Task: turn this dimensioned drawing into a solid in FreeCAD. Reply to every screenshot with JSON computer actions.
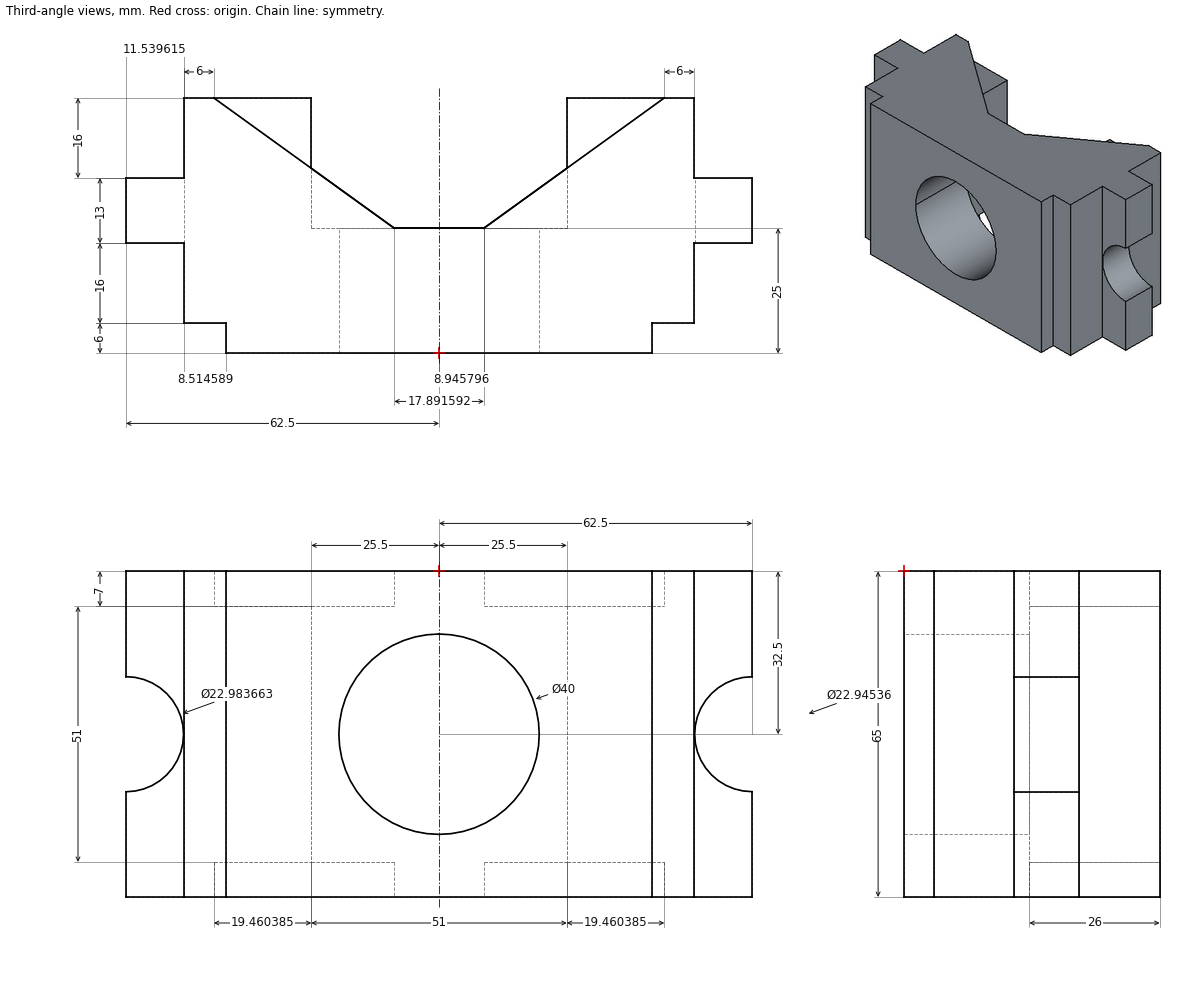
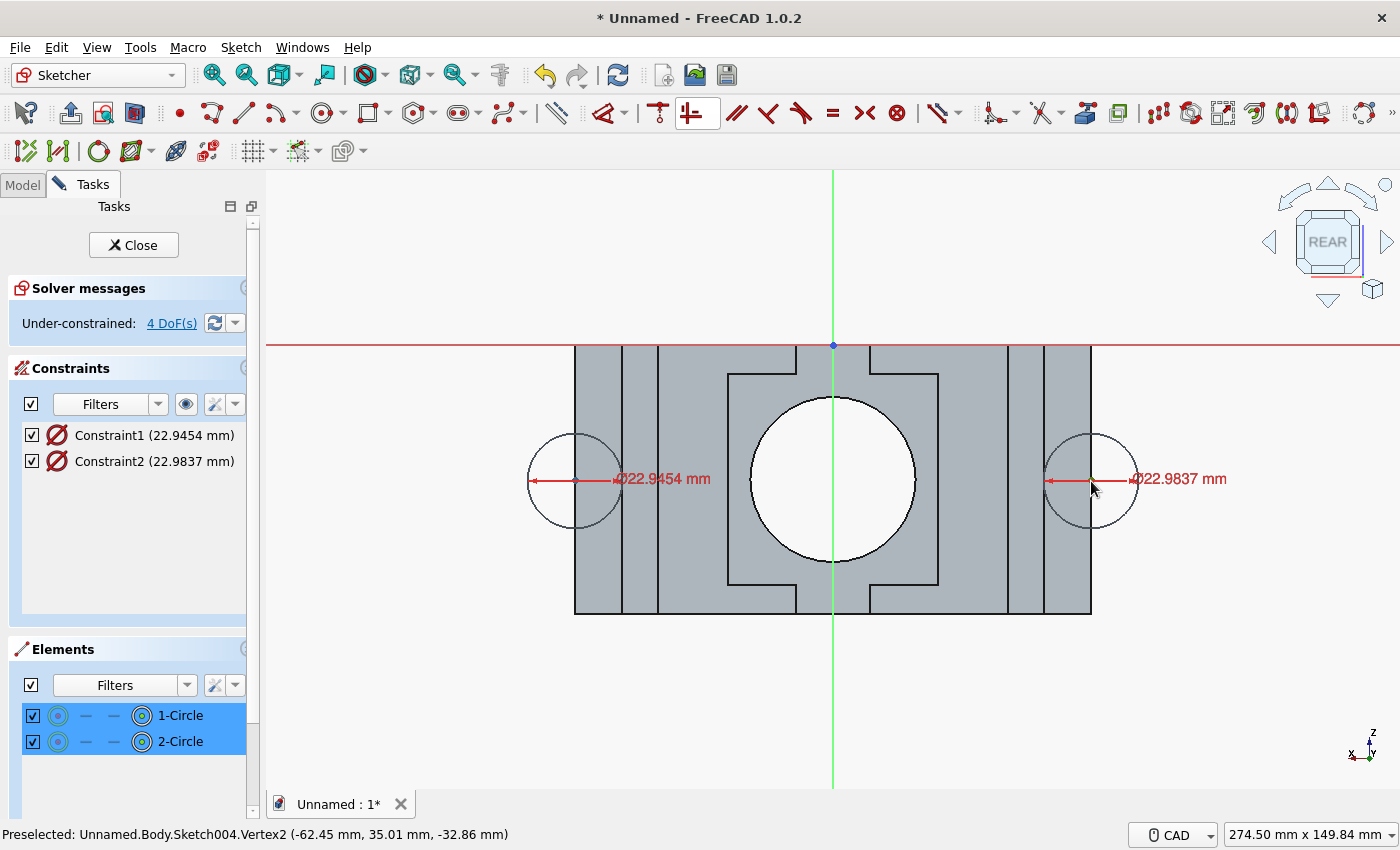
{"action": "left_click", "coordinate": [833, 721]}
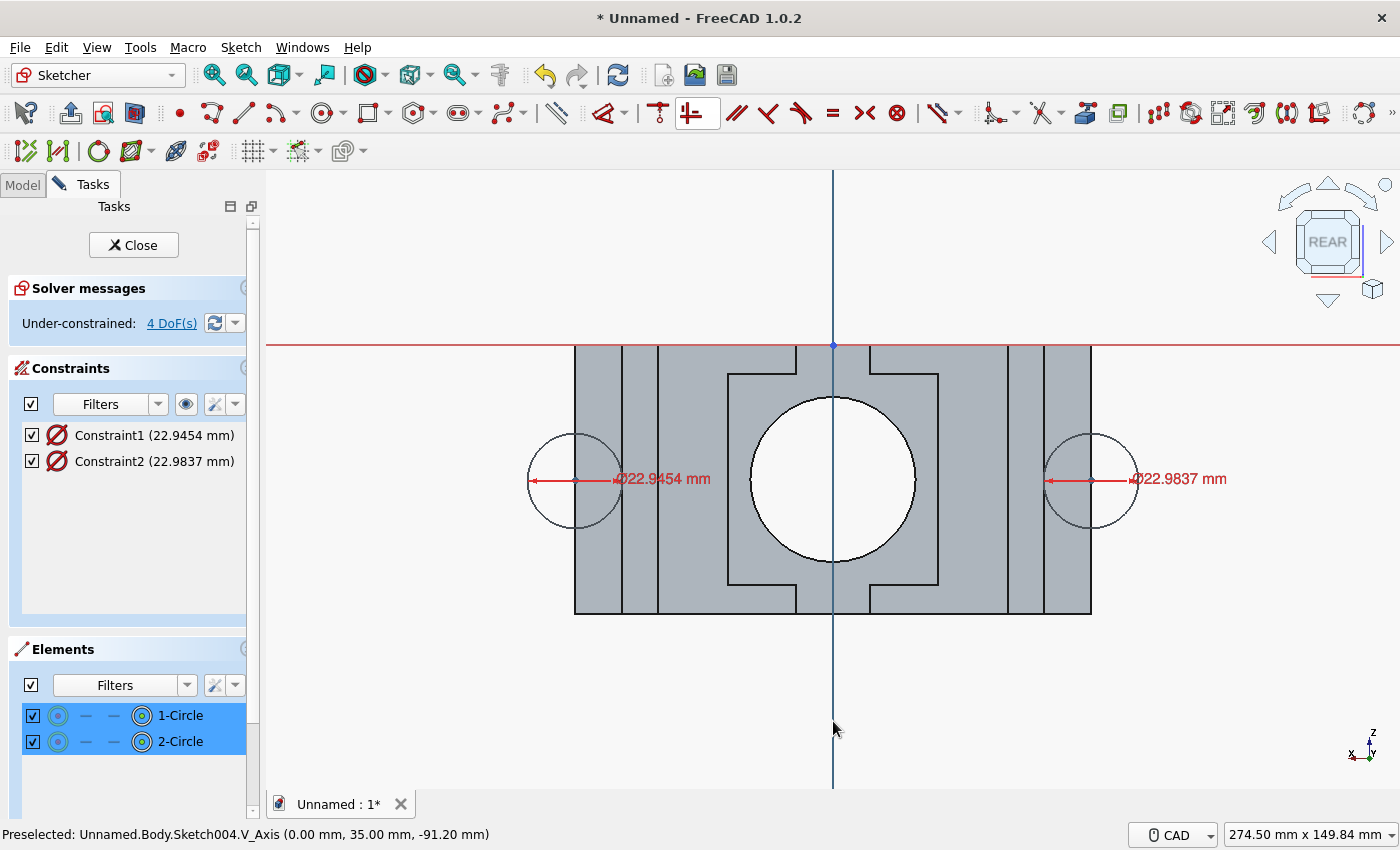
{"action": "left_click", "coordinate": [866, 114]}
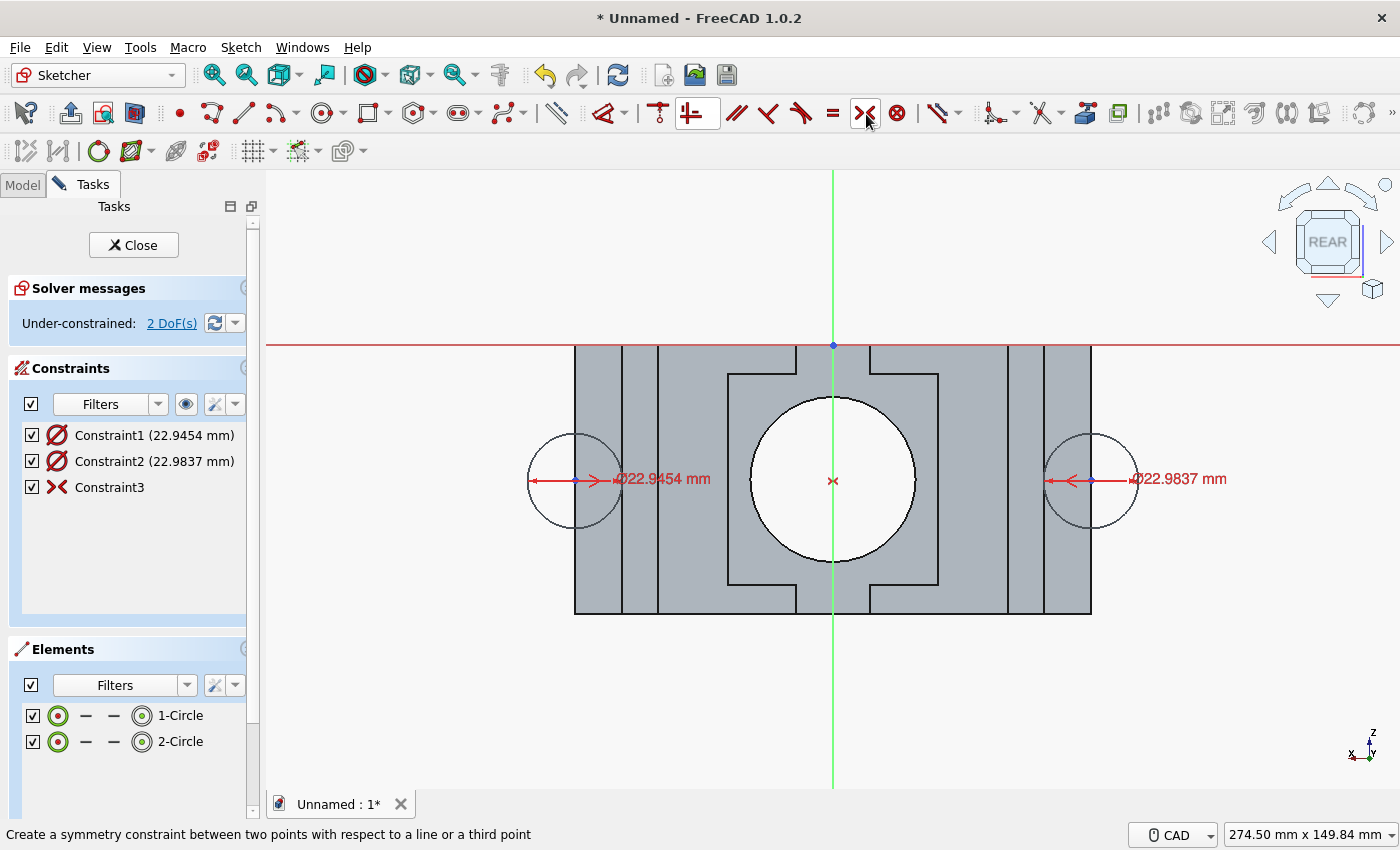
{"action": "left_click", "coordinate": [604, 114]}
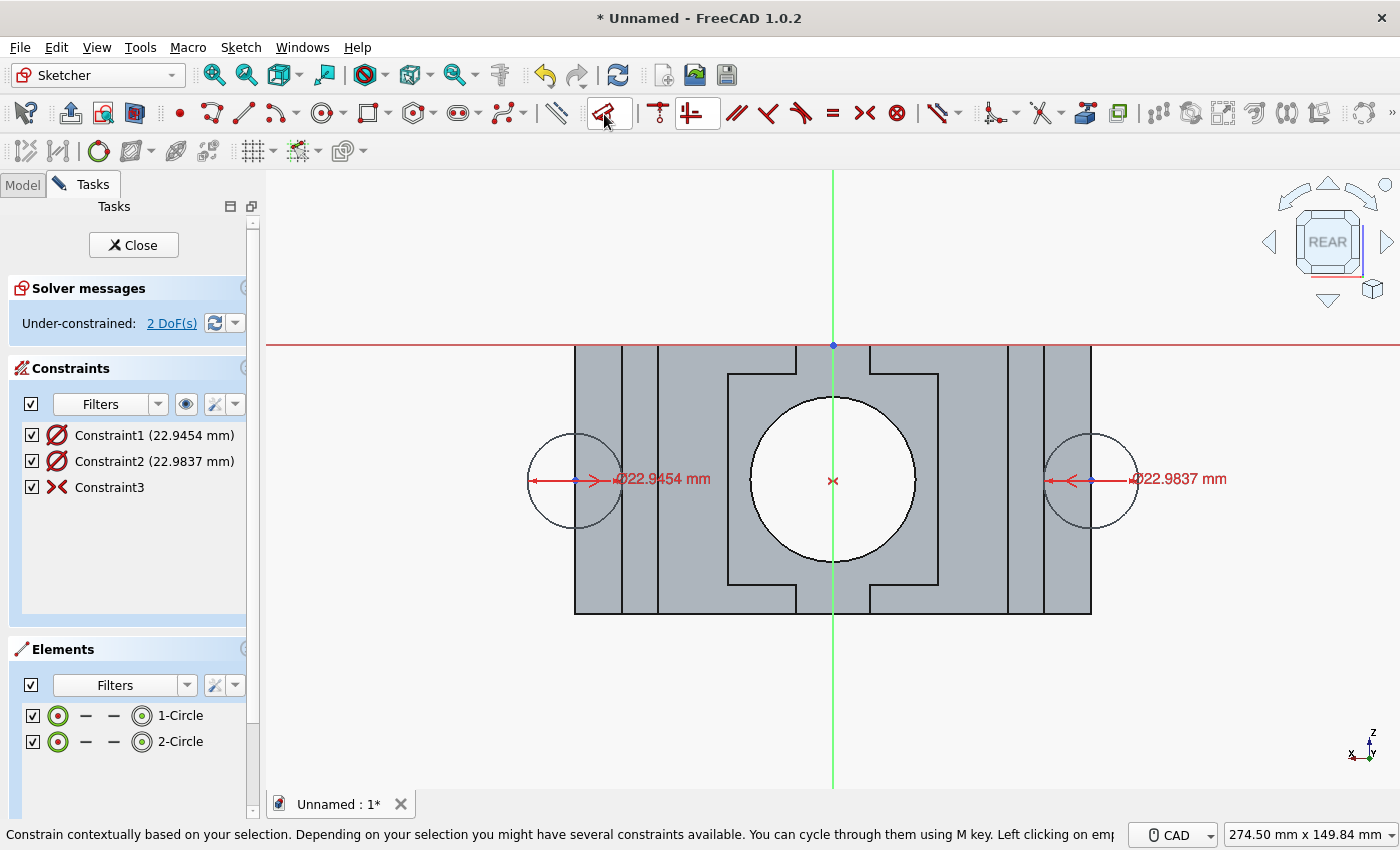
{"action": "left_click", "coordinate": [575, 481]}
{"action": "left_click", "coordinate": [704, 311]}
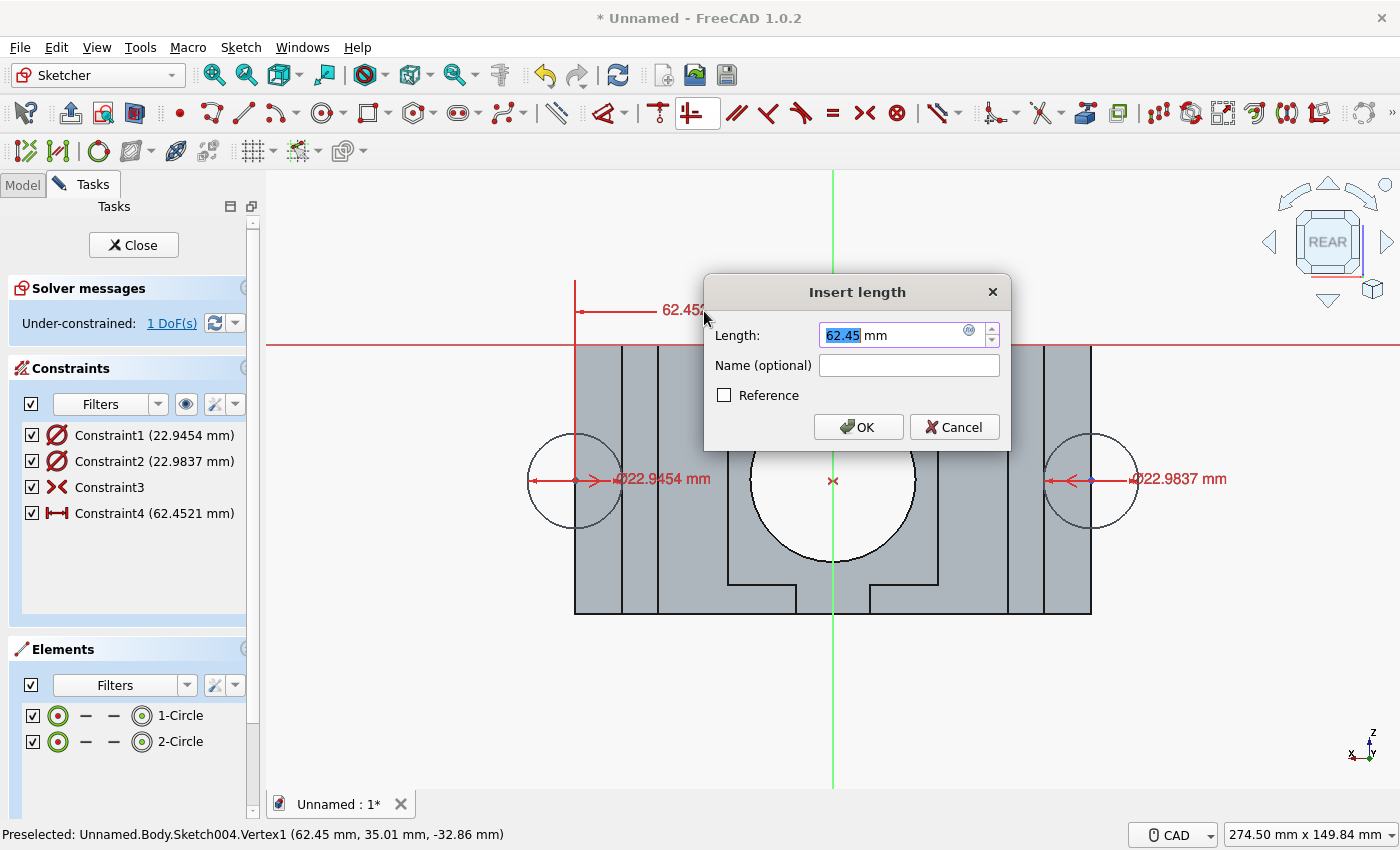
{"action": "type", "text": "62.5"}
{"action": "key", "text": "Return"}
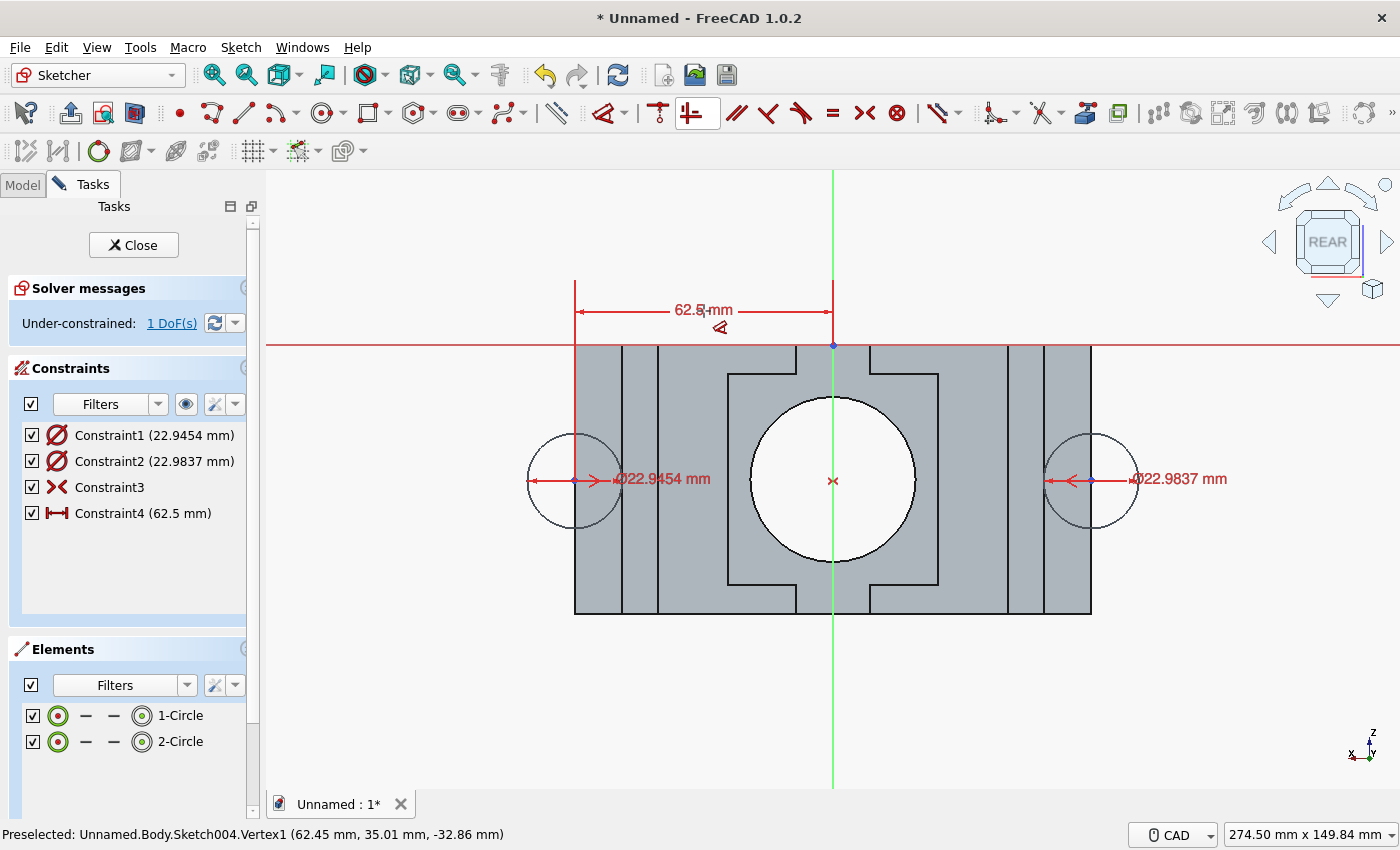
{"action": "left_click", "coordinate": [575, 481]}
{"action": "left_click", "coordinate": [541, 413]}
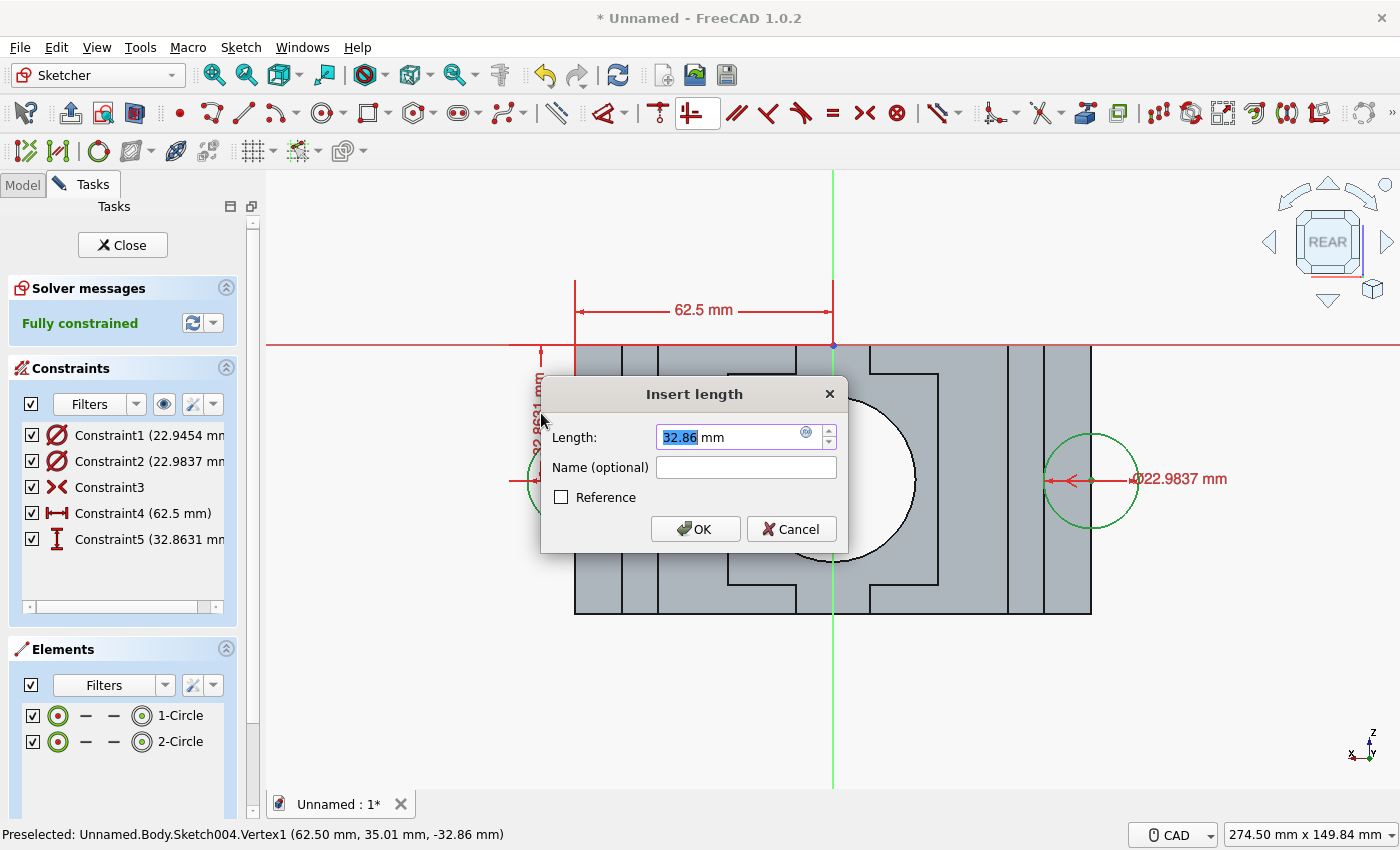
{"action": "type", "text": "32.5"}
{"action": "key", "text": "Return"}
{"action": "key", "text": "Escape"}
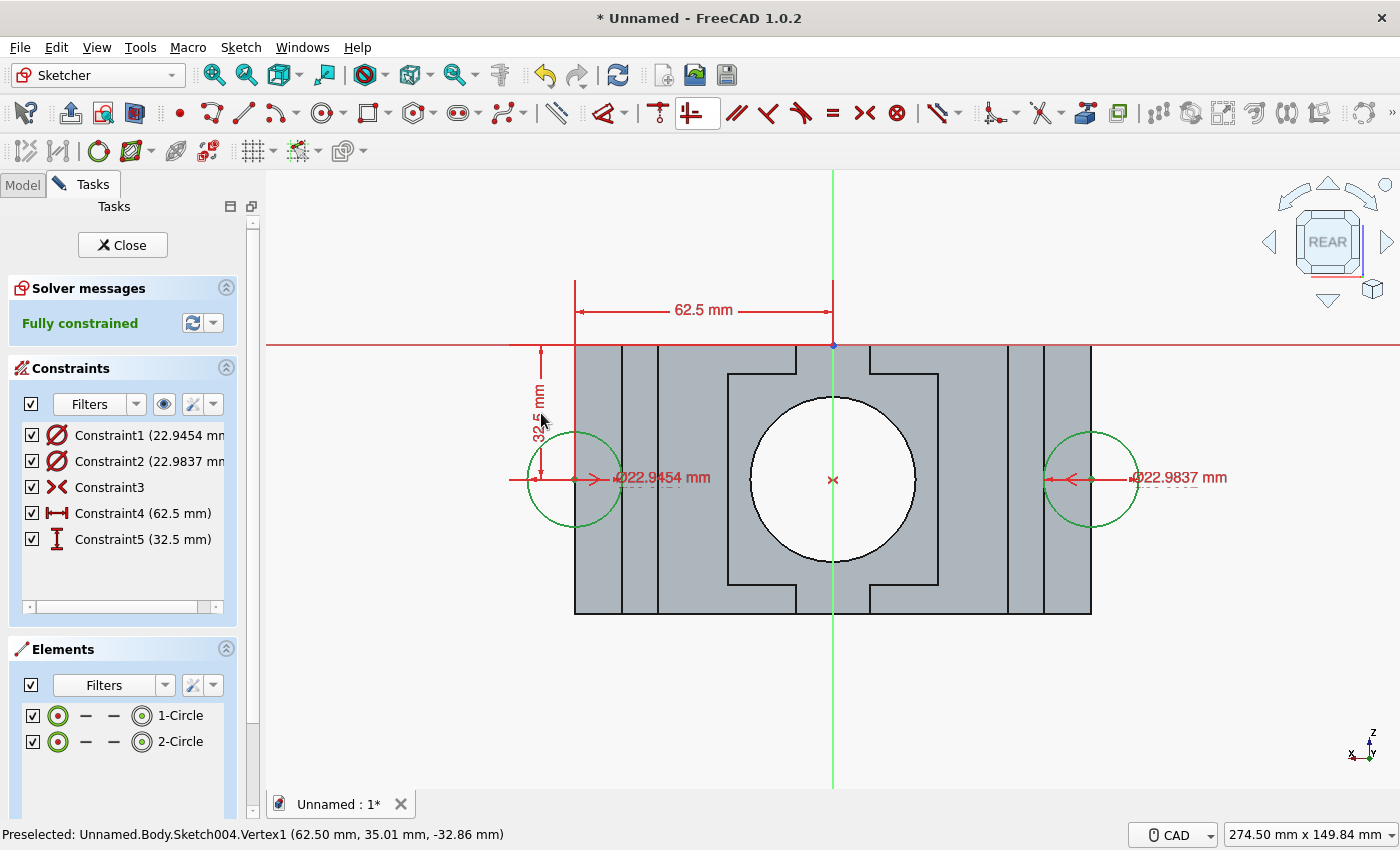
{"action": "left_click", "coordinate": [123, 245]}